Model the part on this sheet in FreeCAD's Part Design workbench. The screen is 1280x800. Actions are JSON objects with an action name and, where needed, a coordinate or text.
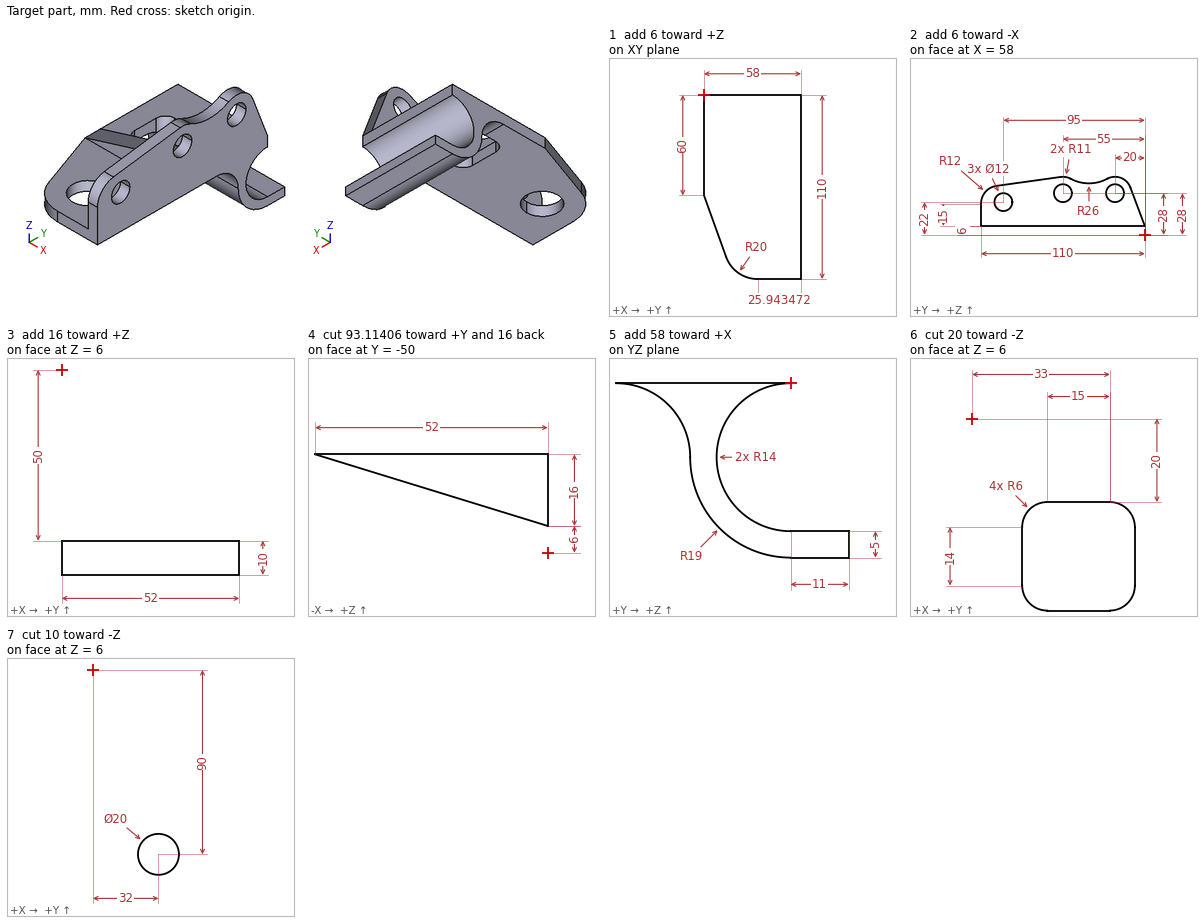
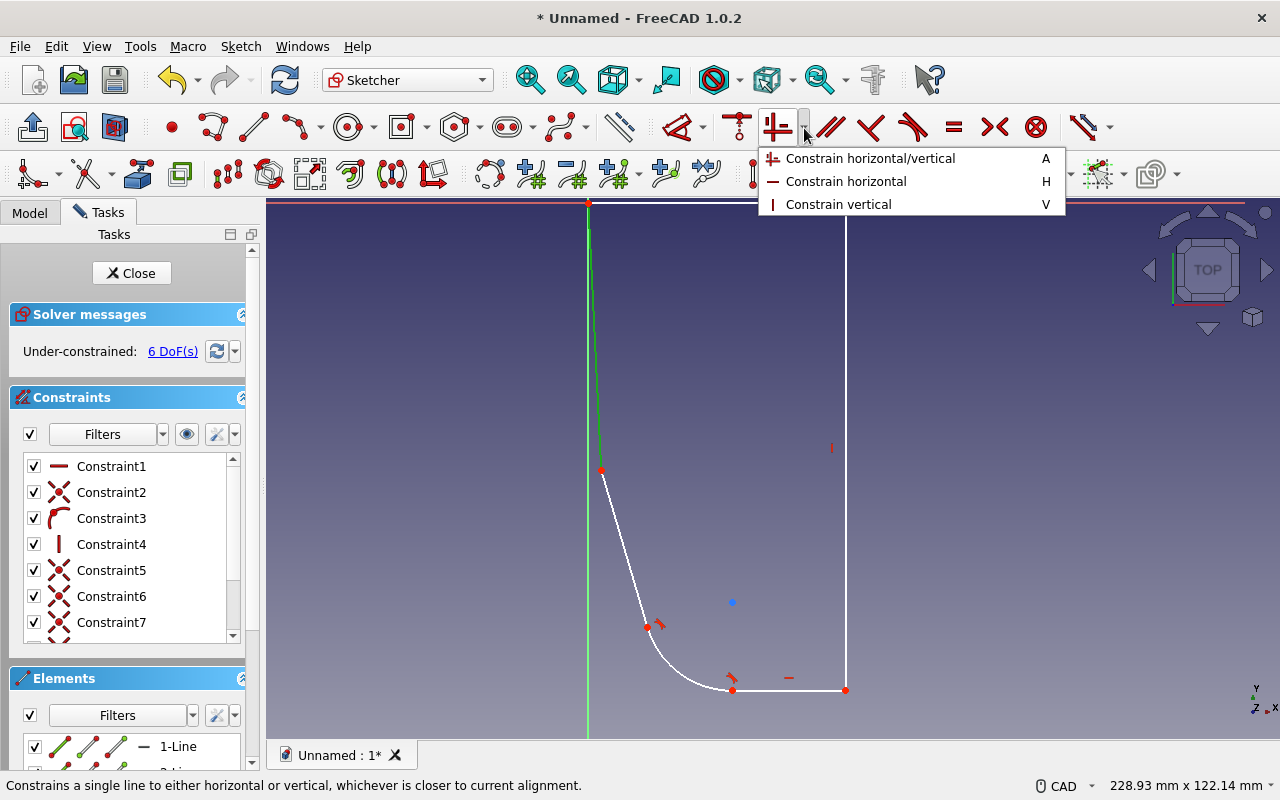
{"action": "left_click", "coordinate": [912, 204]}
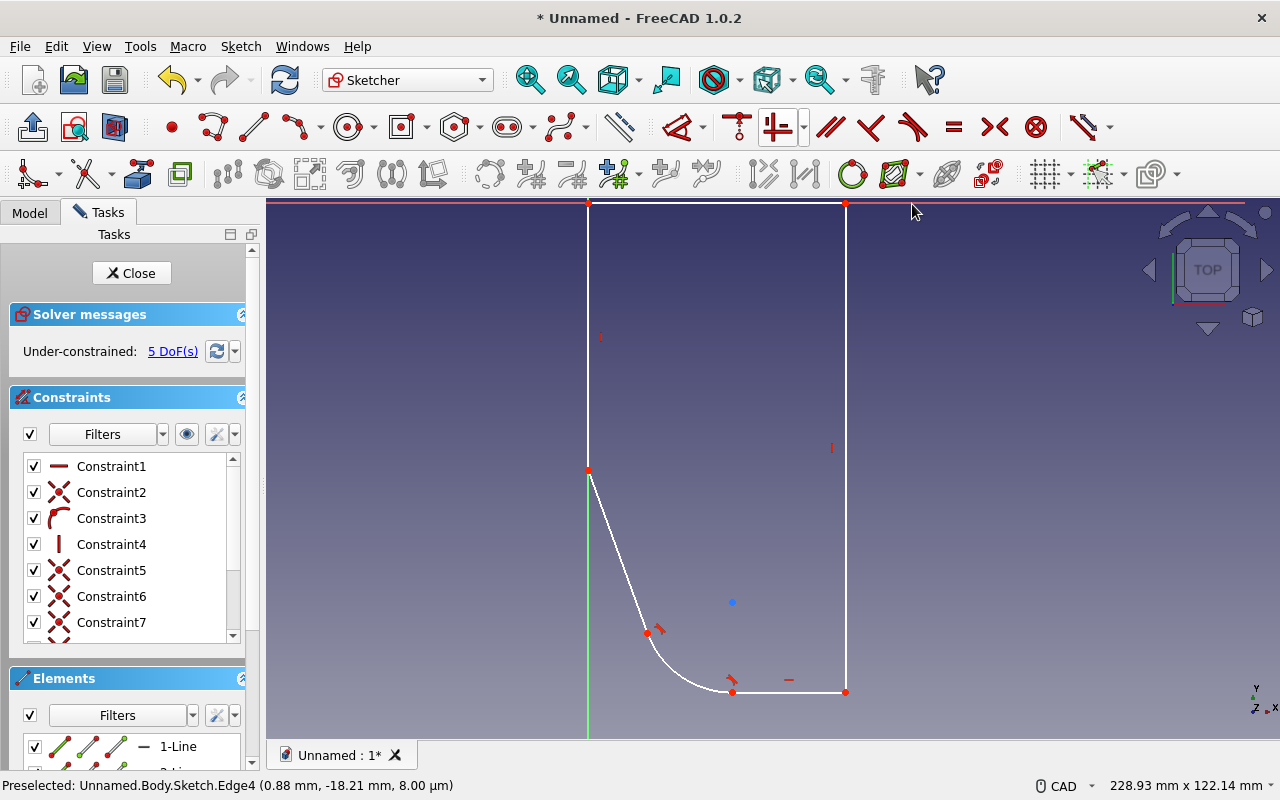
{"action": "left_click", "coordinate": [676, 128]}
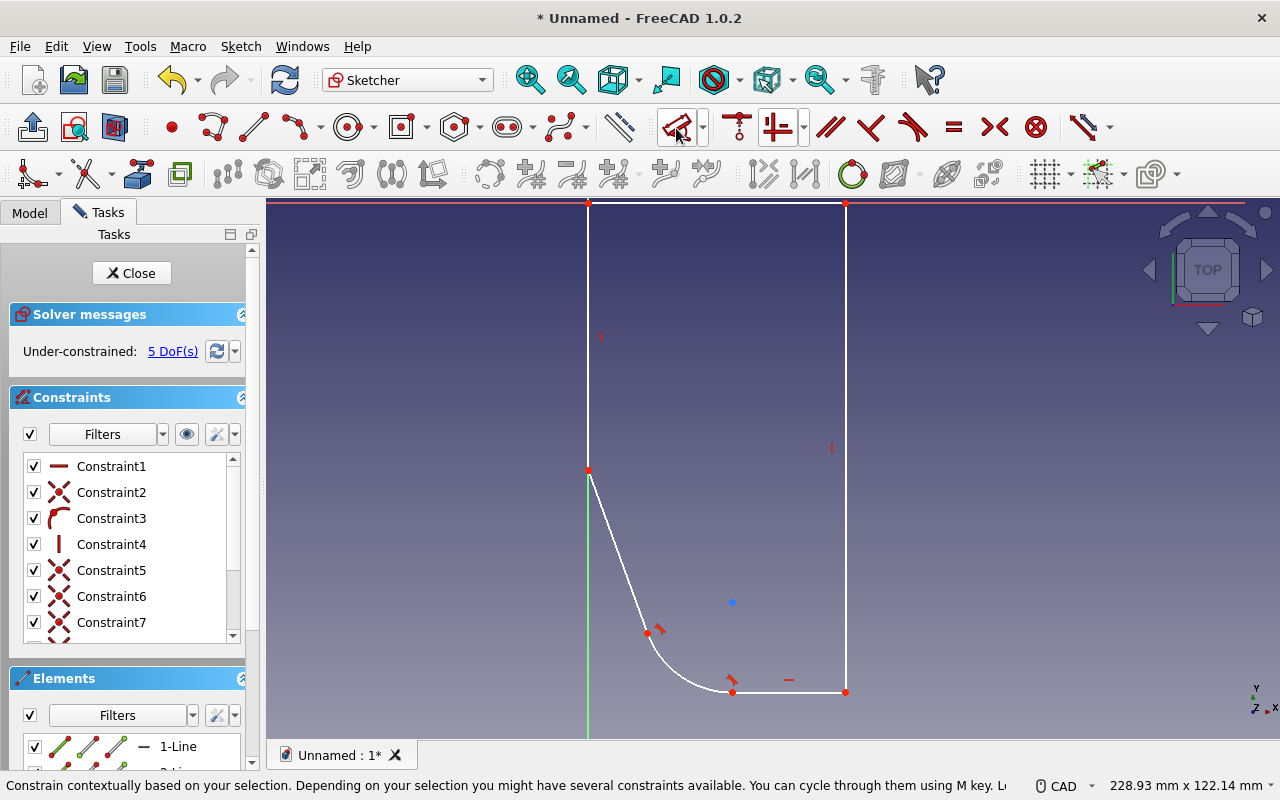
{"action": "left_click", "coordinate": [664, 661]}
{"action": "left_click", "coordinate": [640, 682]}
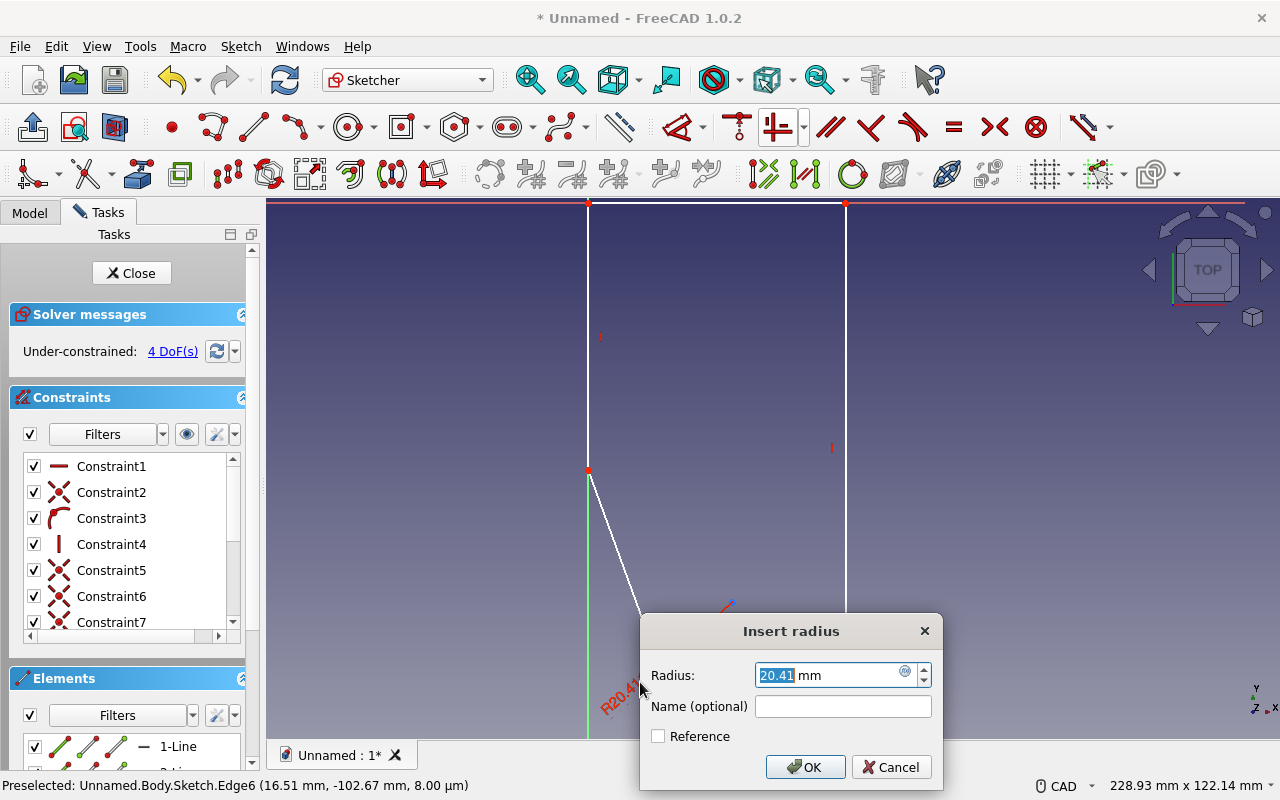
{"action": "type", "text": "20"}
{"action": "key", "text": "Return"}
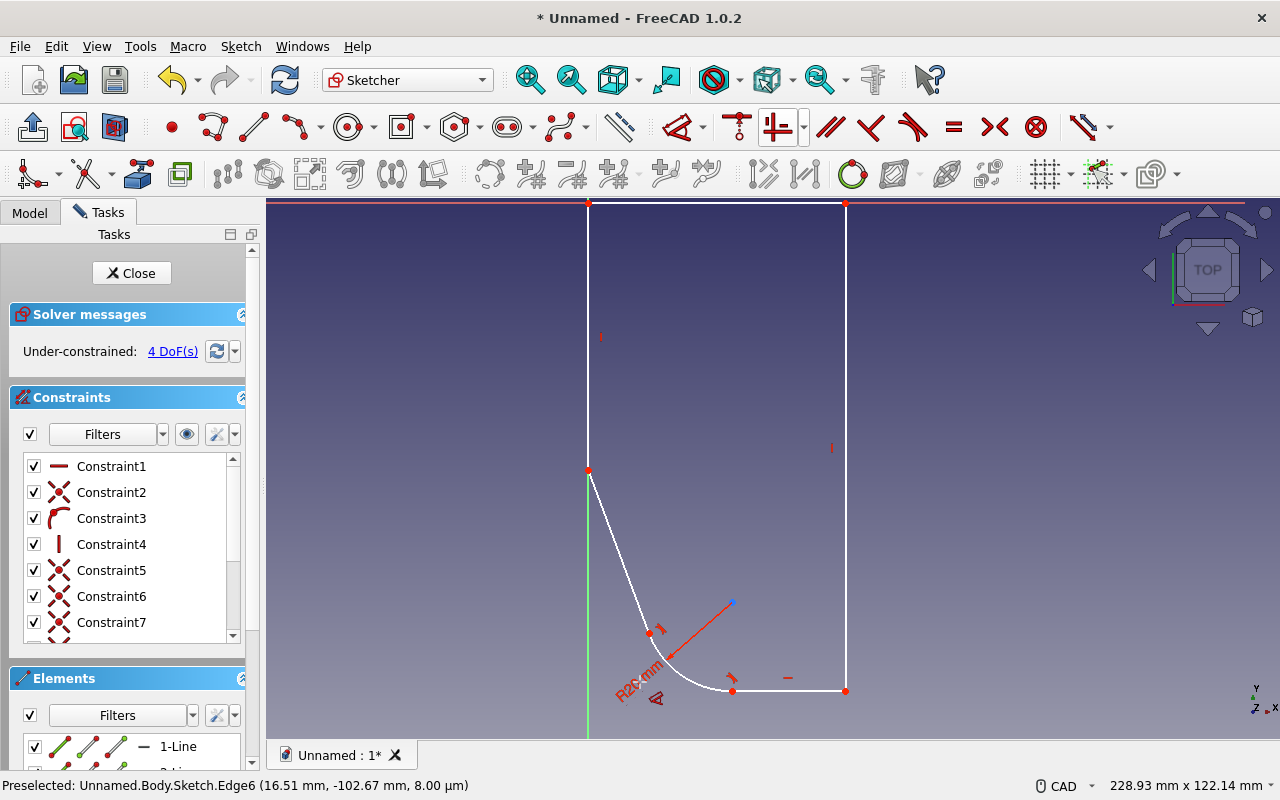
{"action": "scroll", "coordinate": [680, 512], "scroll_direction": "down", "scroll_amount": 2}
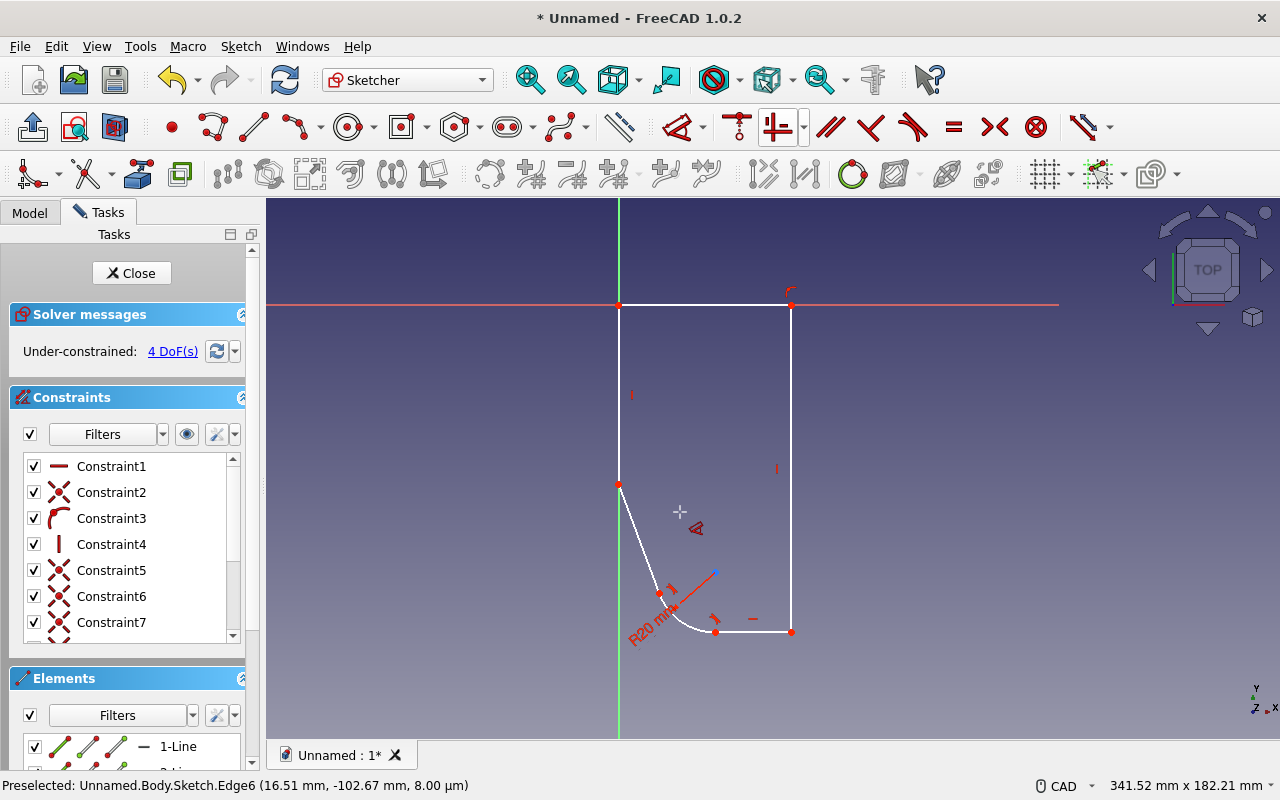
{"action": "left_click", "coordinate": [740, 305]}
{"action": "left_click", "coordinate": [705, 271]}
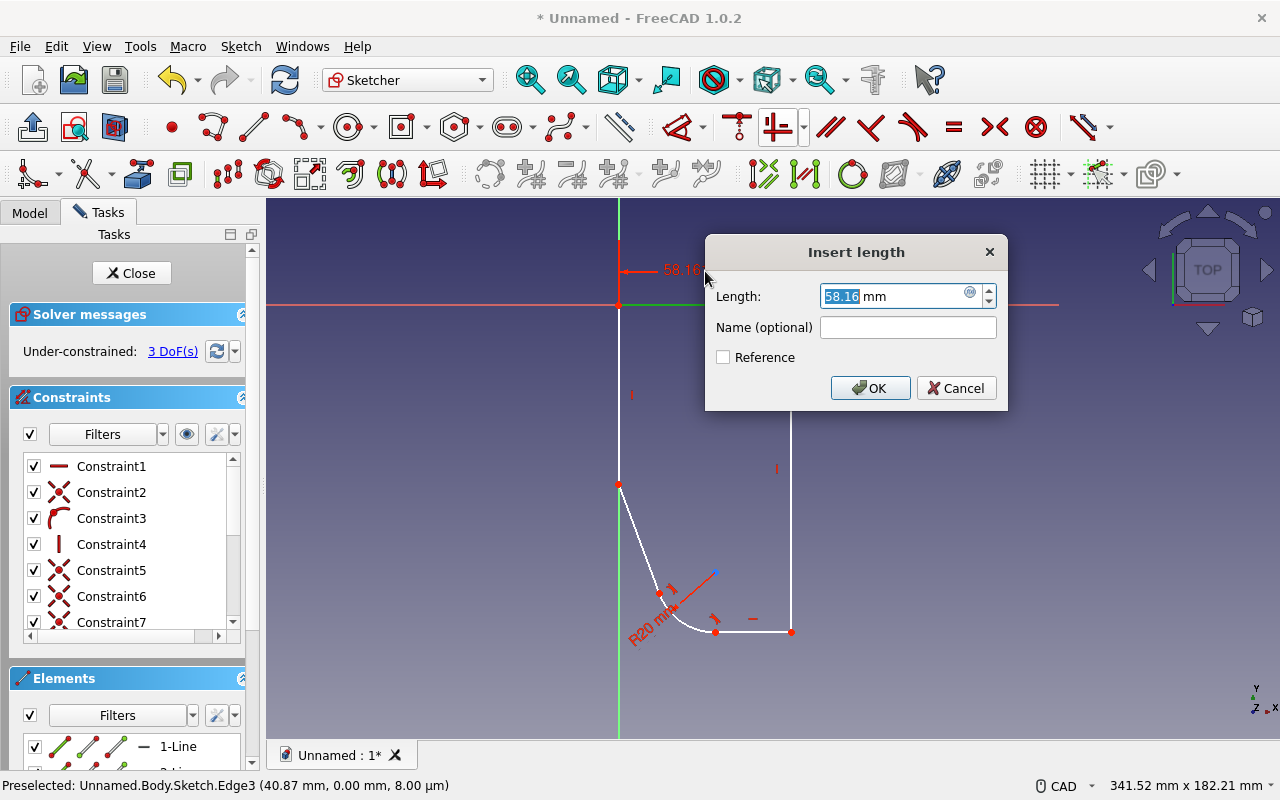
{"action": "type", "text": "58"}
{"action": "key", "text": "Return"}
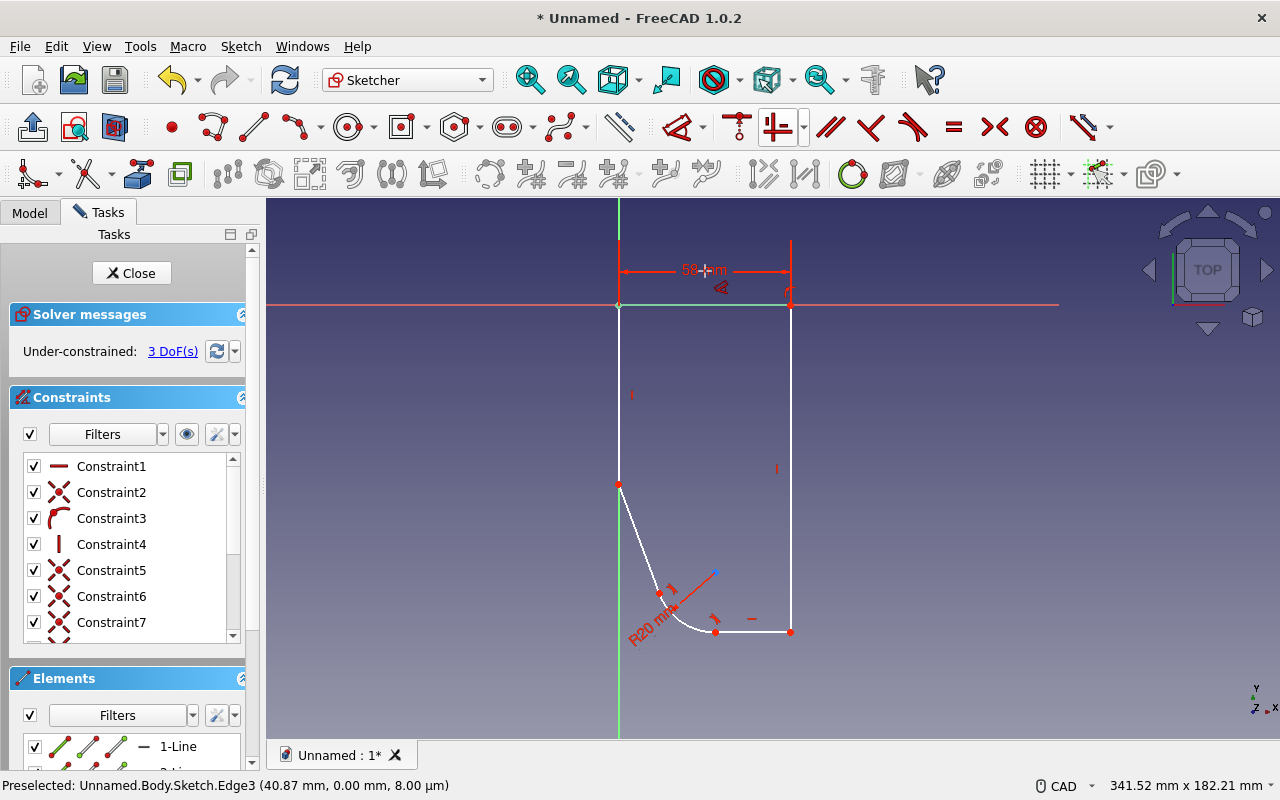
{"action": "left_click", "coordinate": [619, 359]}
{"action": "left_click", "coordinate": [585, 395]}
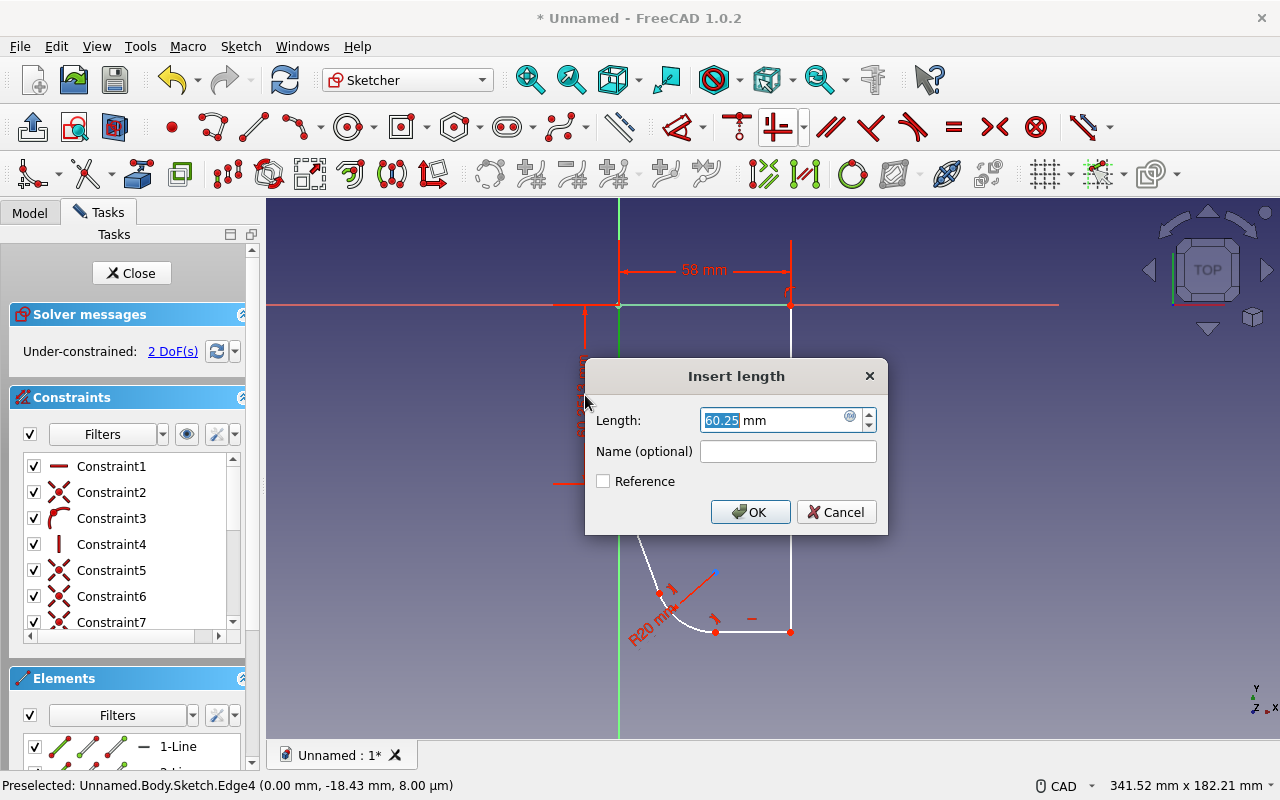
{"action": "type", "text": "60"}
{"action": "key", "text": "Return"}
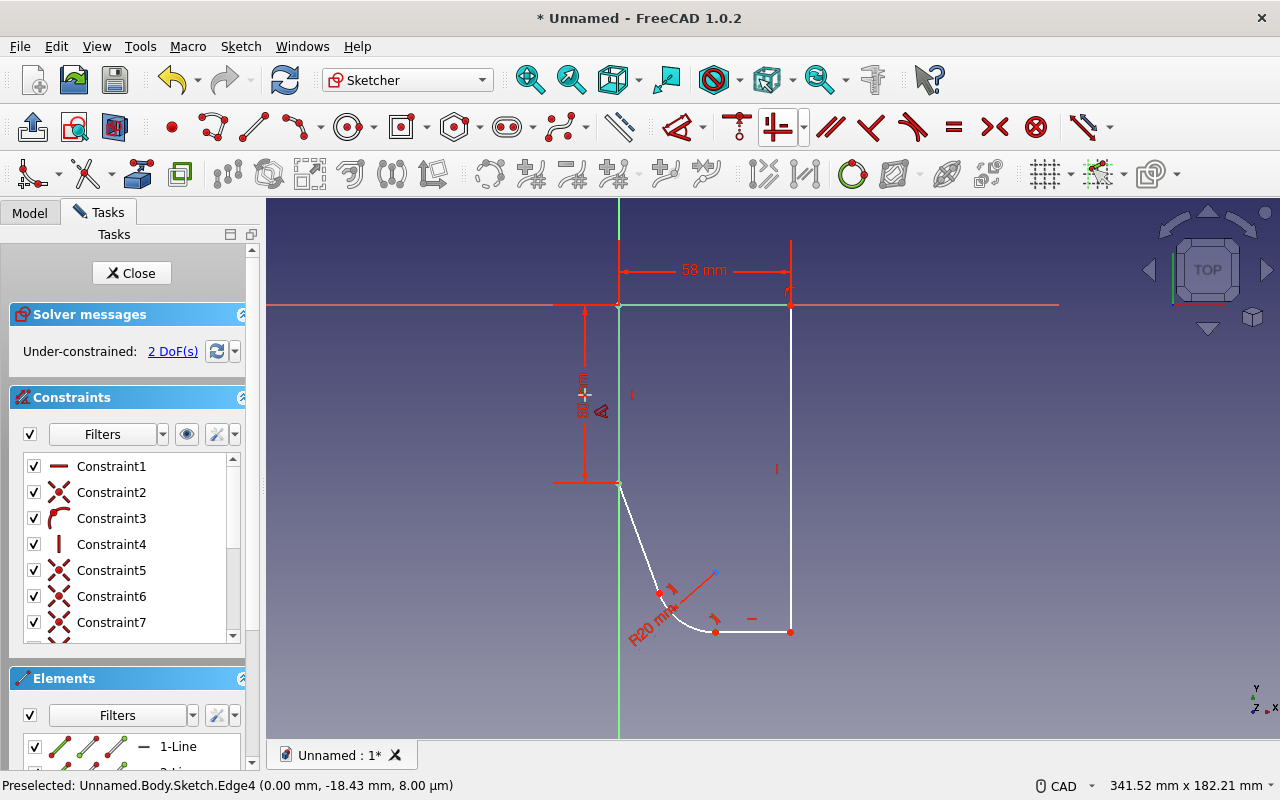
{"action": "left_click", "coordinate": [791, 534]}
{"action": "left_click", "coordinate": [825, 469]}